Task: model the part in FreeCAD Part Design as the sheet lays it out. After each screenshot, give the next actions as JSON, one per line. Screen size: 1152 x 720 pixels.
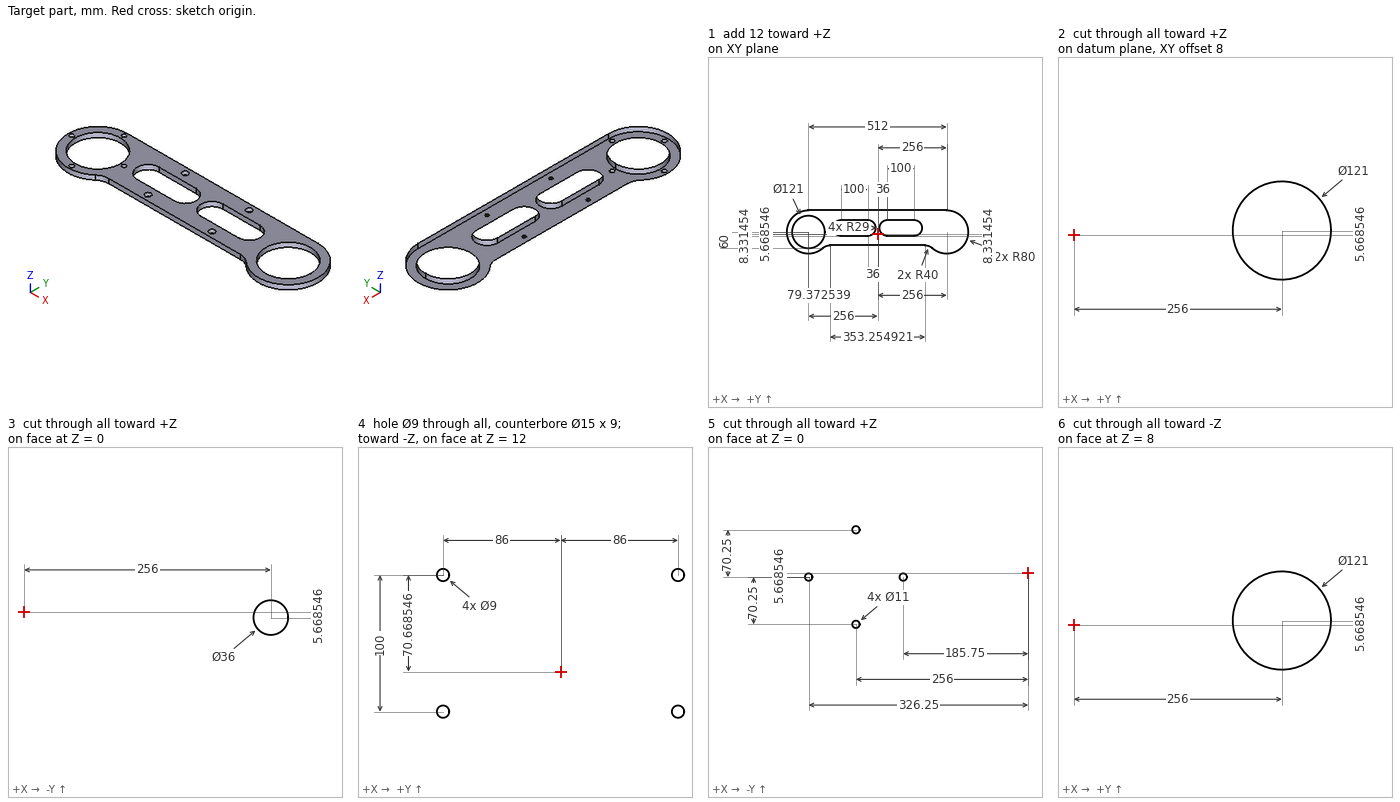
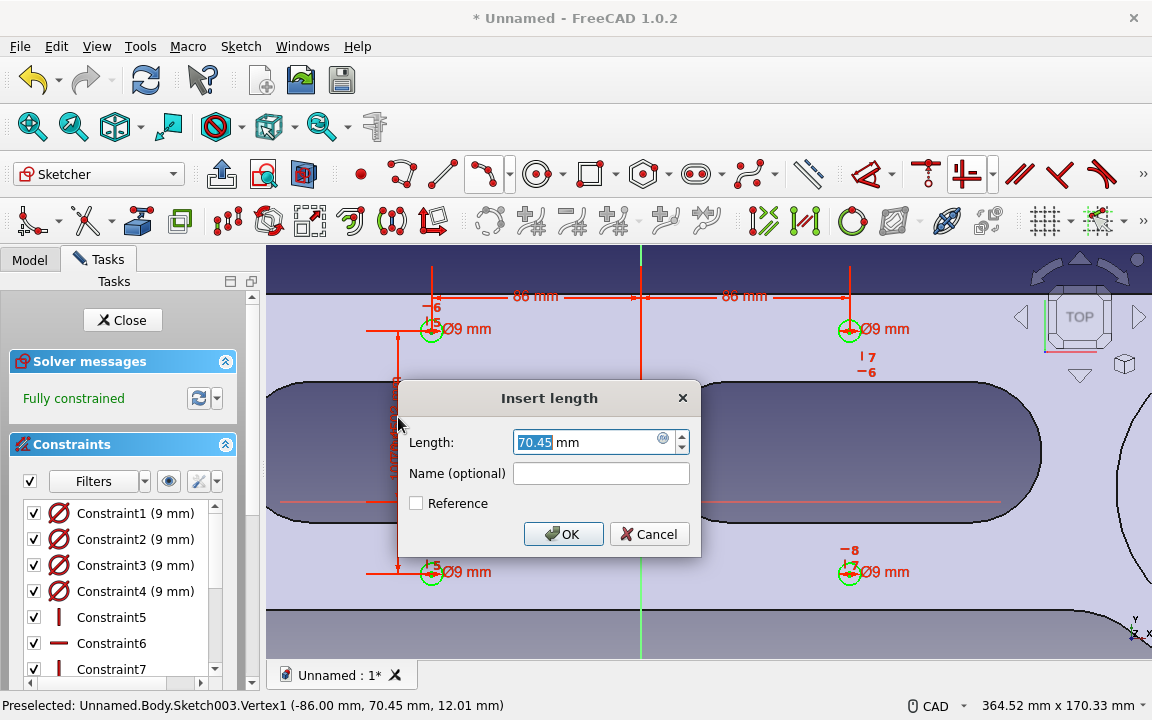
{"action": "type", "text": "70.668546"}
{"action": "key", "text": "Return"}
{"action": "key", "text": "Escape"}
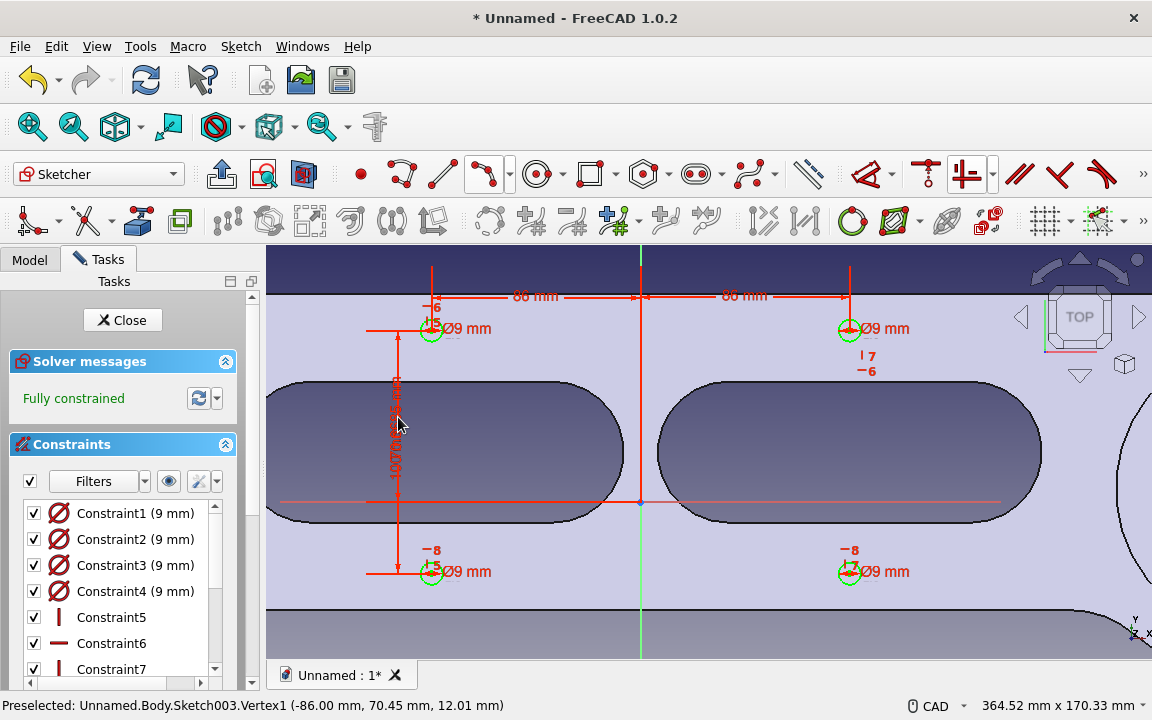
{"action": "left_click", "coordinate": [123, 320]}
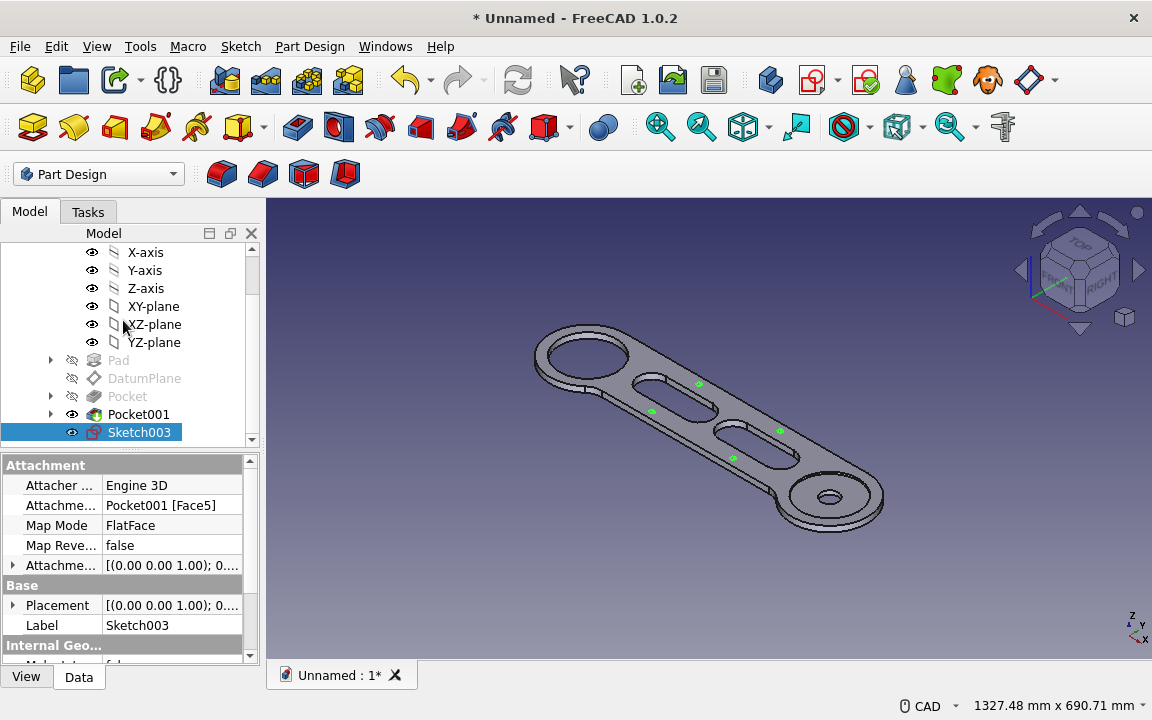
{"action": "left_click", "coordinate": [339, 128]}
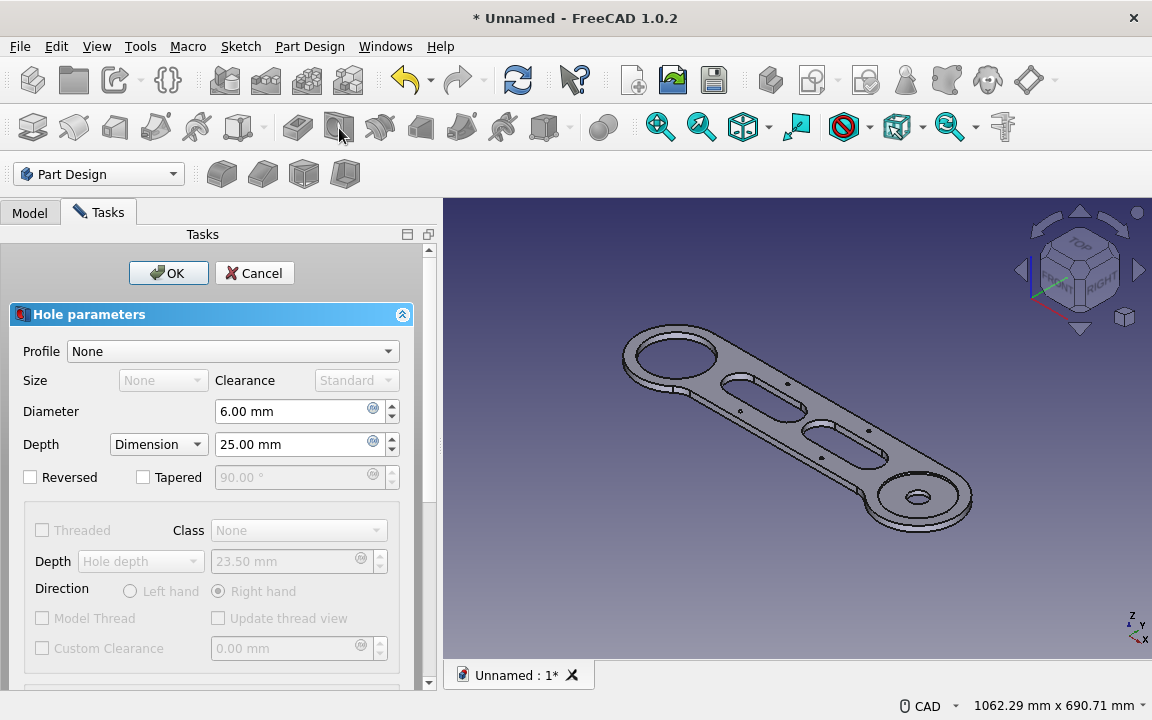
{"action": "triple_click", "coordinate": [300, 412]}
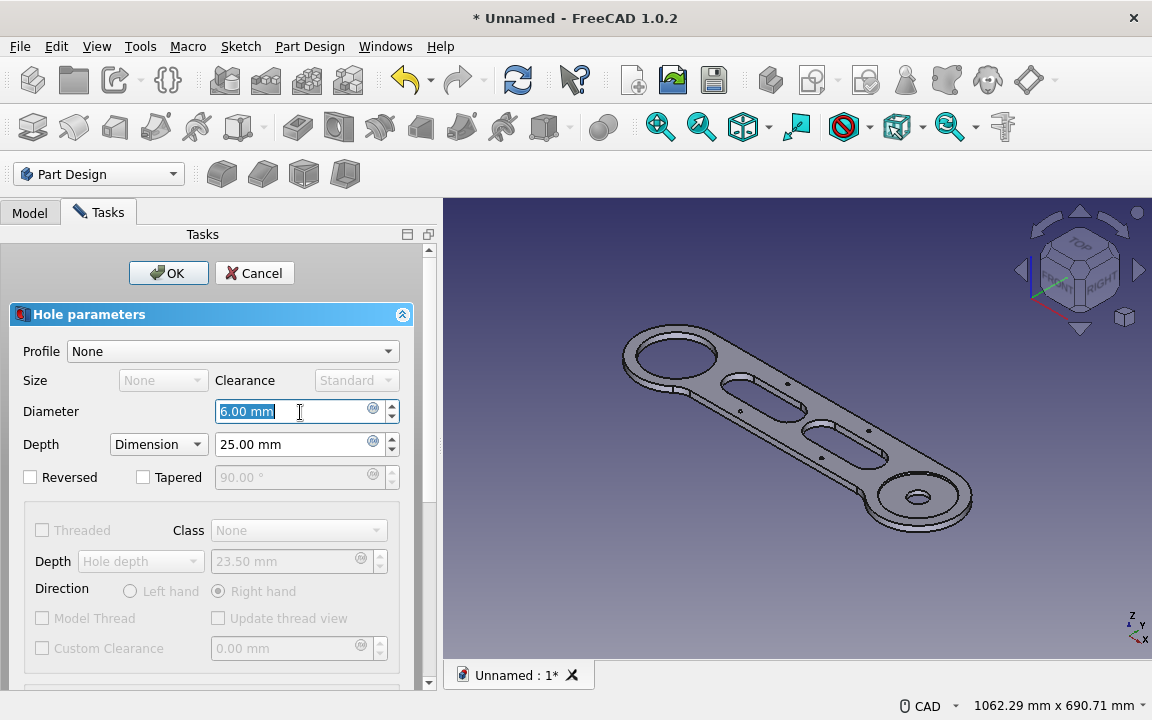
{"action": "type", "text": "9"}
{"action": "key", "text": "Tab"}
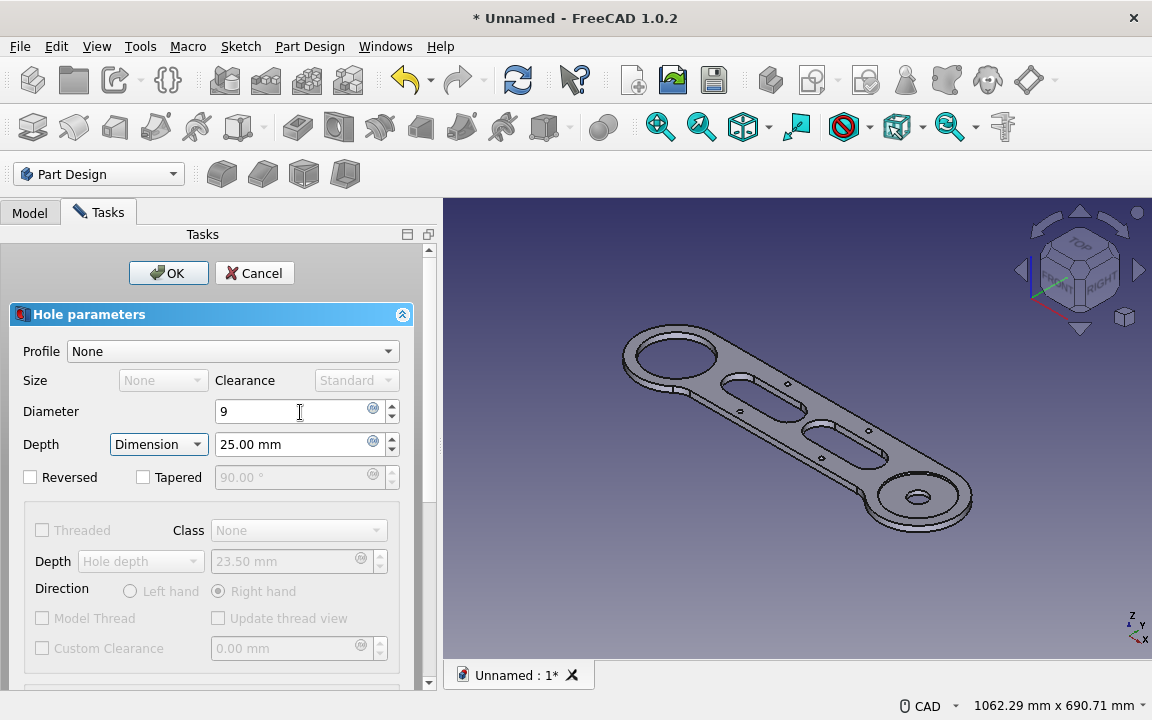
{"action": "left_click", "coordinate": [160, 444]}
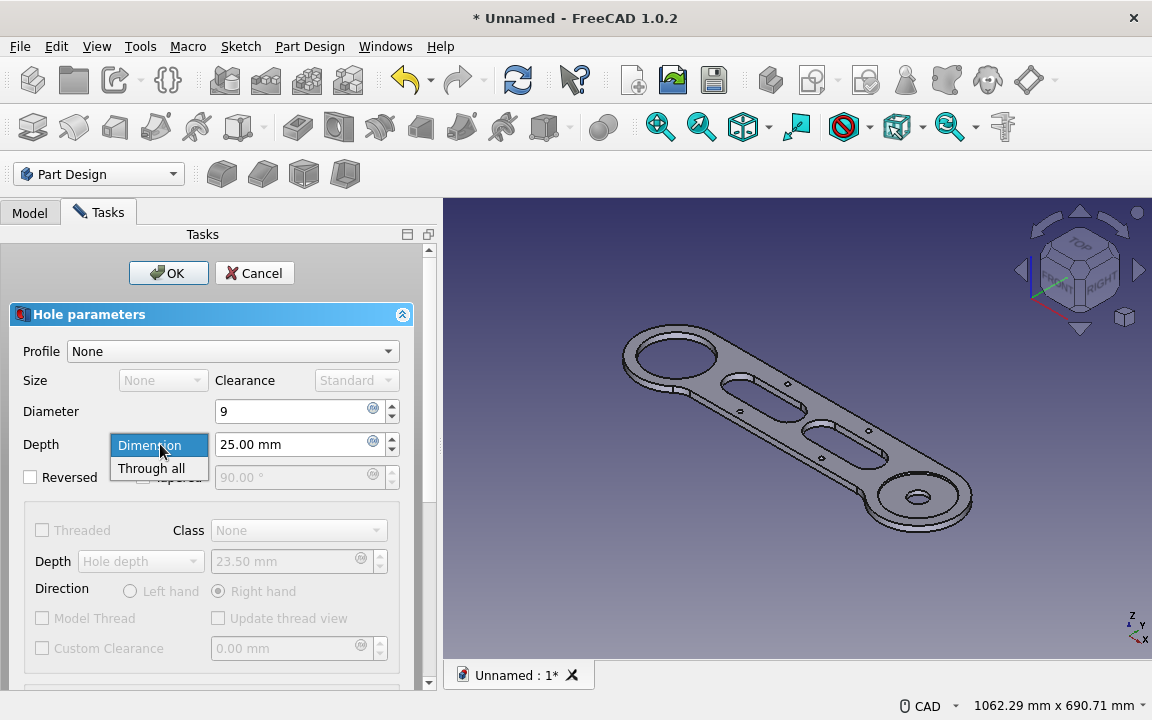
{"action": "left_click", "coordinate": [158, 468]}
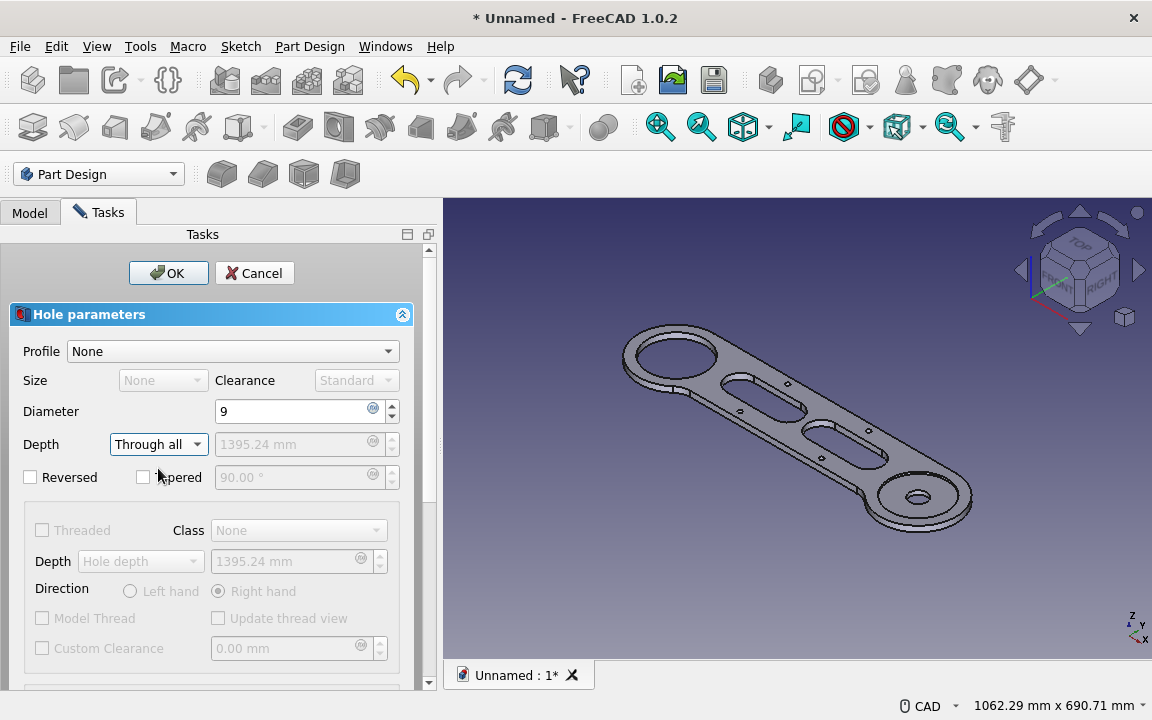
{"action": "scroll", "coordinate": [429, 467], "scroll_direction": "down", "scroll_amount": 2}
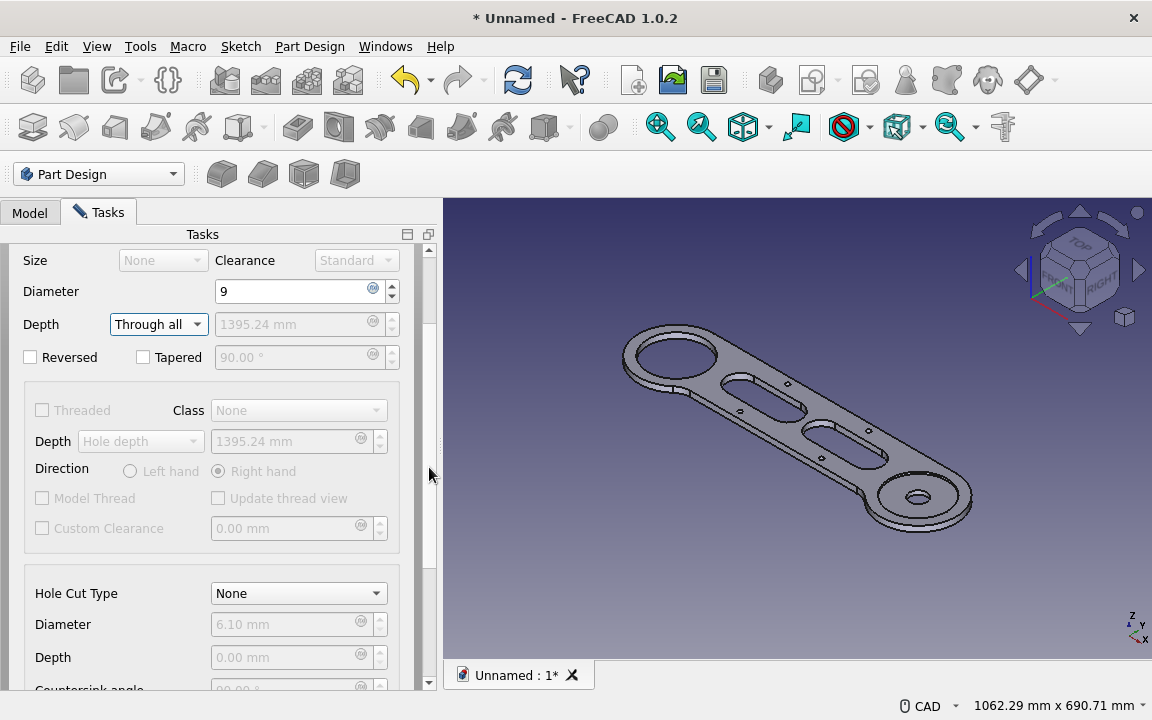
{"action": "left_click", "coordinate": [300, 594]}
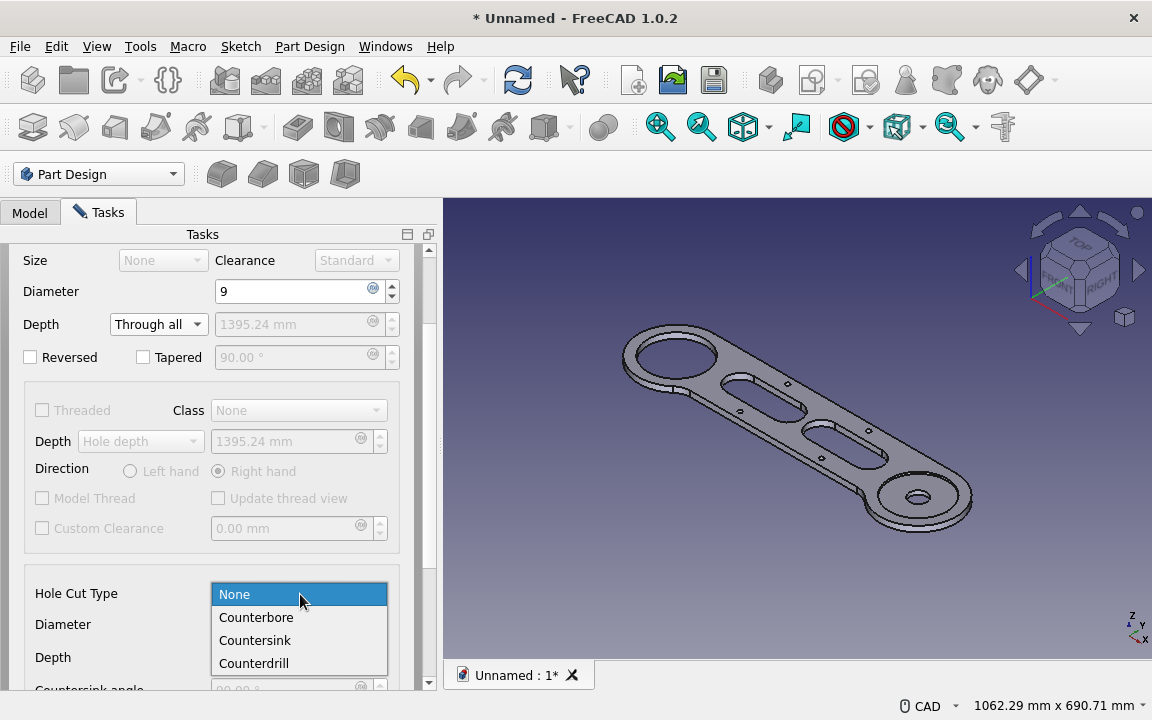
{"action": "left_click", "coordinate": [298, 618]}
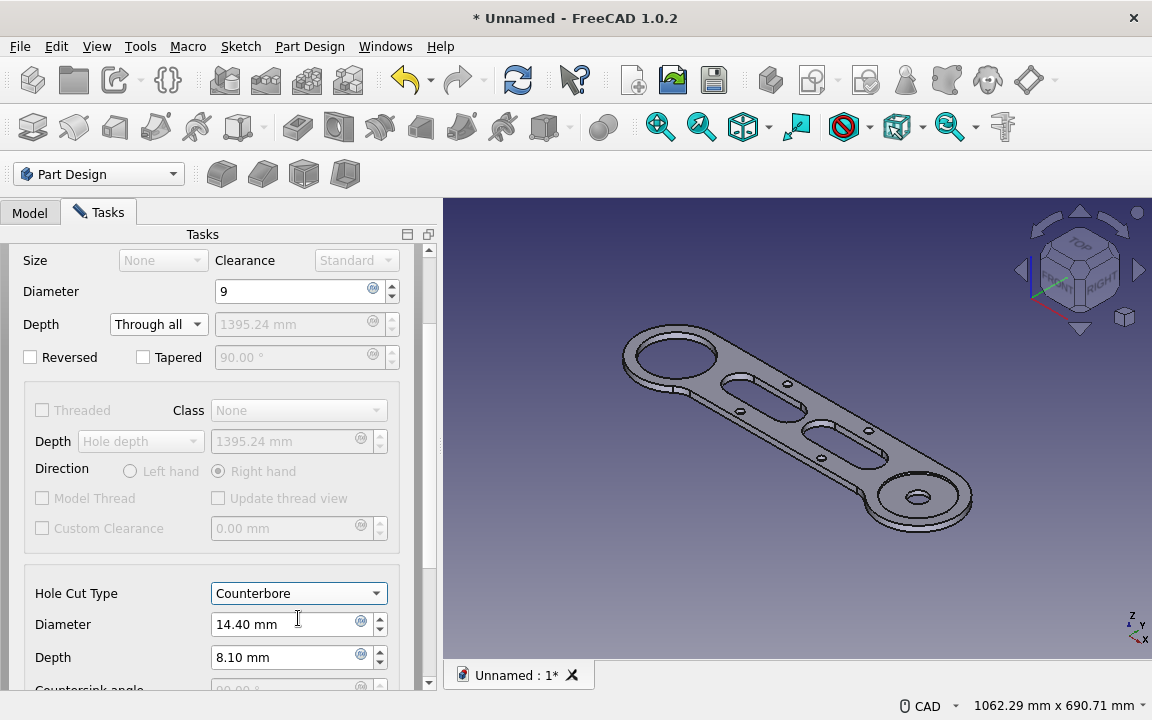
{"action": "triple_click", "coordinate": [292, 624]}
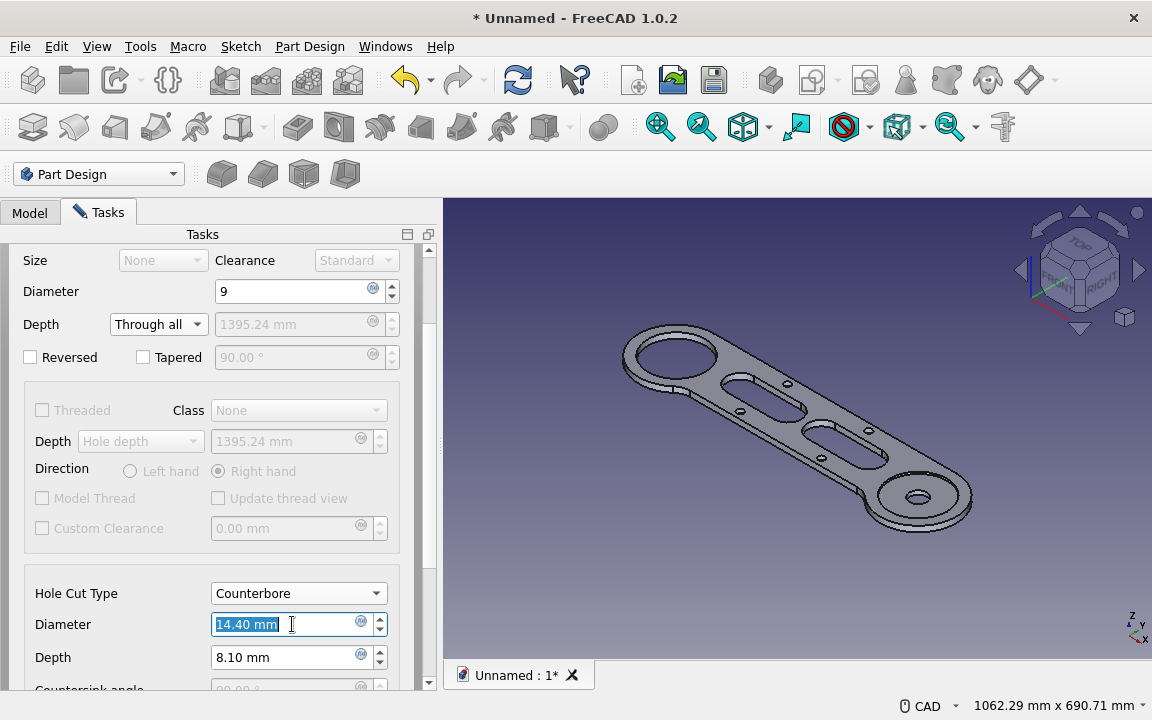
{"action": "type", "text": "15"}
{"action": "key", "text": "Tab"}